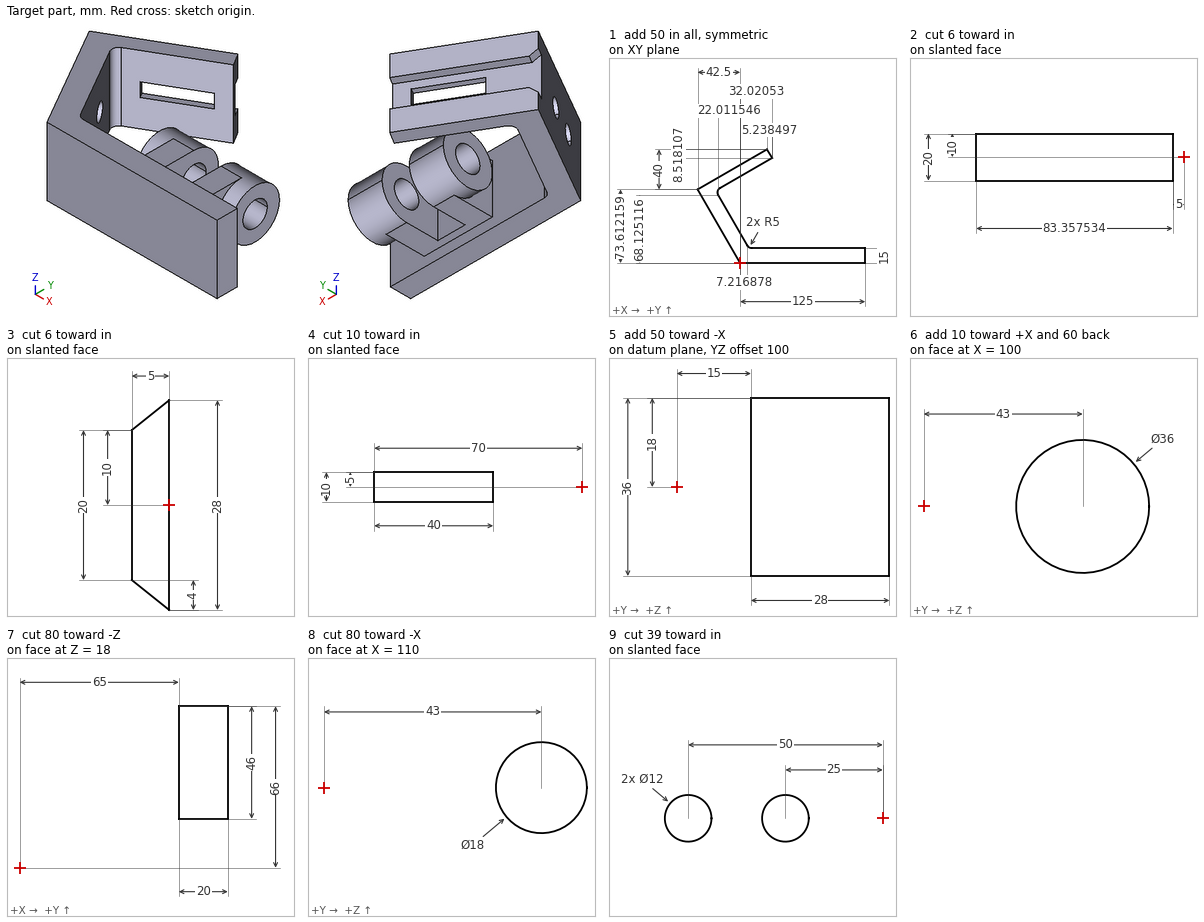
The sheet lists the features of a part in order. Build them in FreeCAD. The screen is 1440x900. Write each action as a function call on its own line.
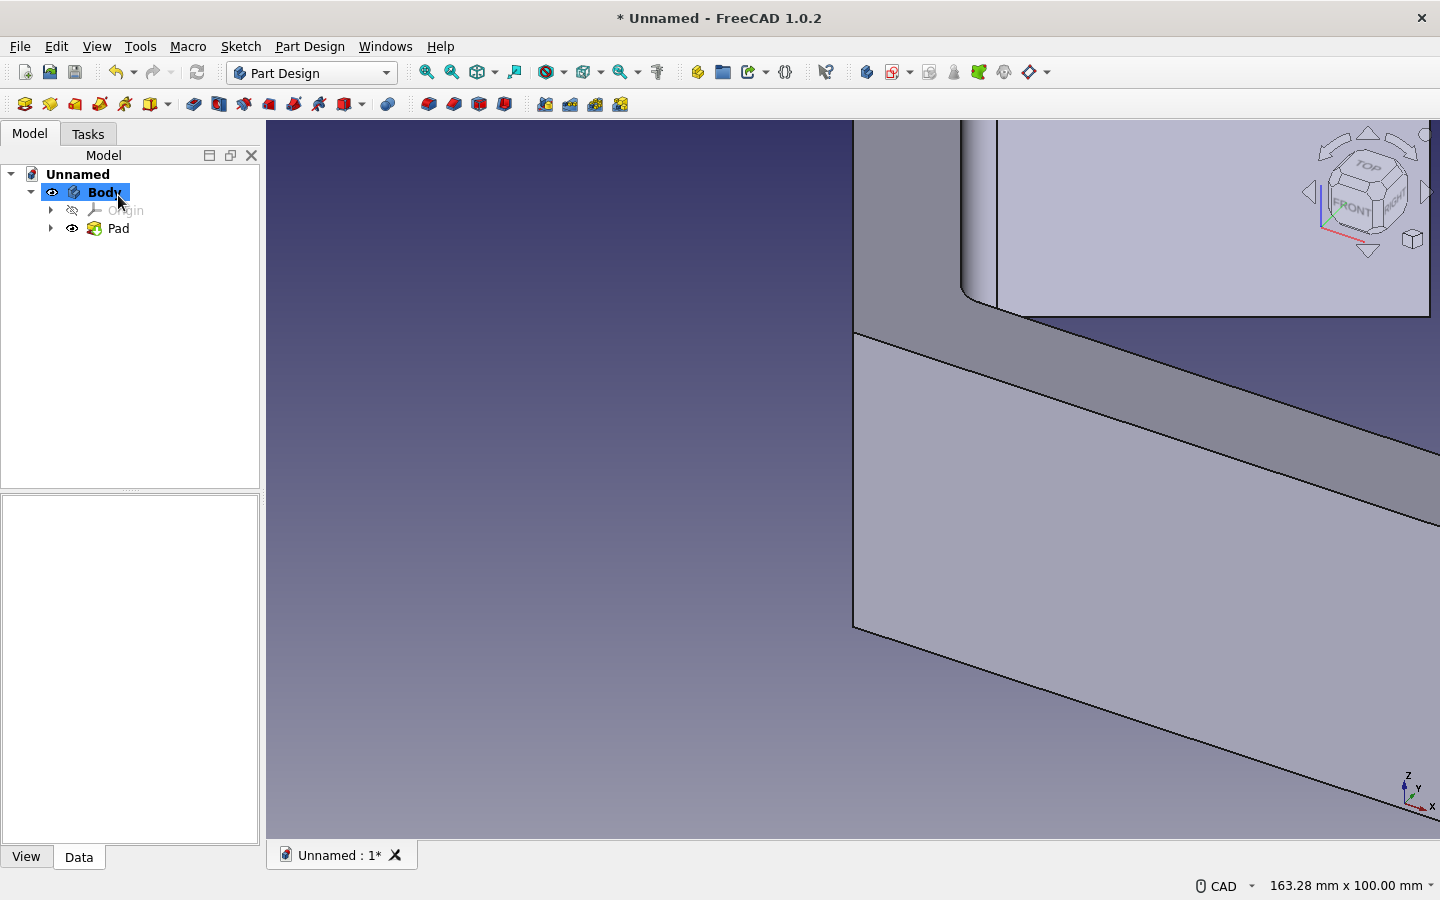
key(v)
key(f)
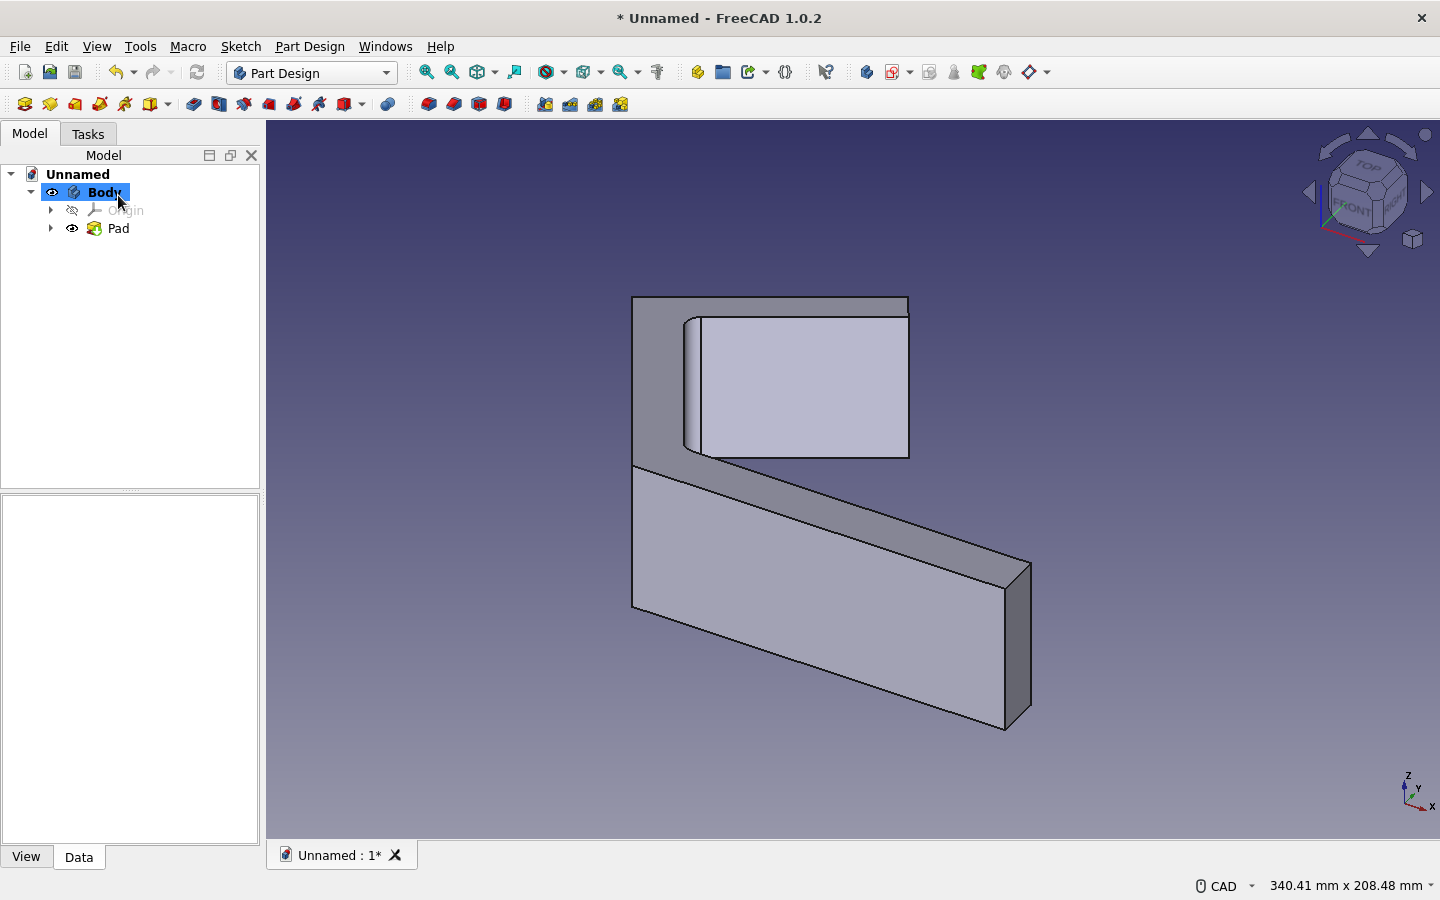
key(4)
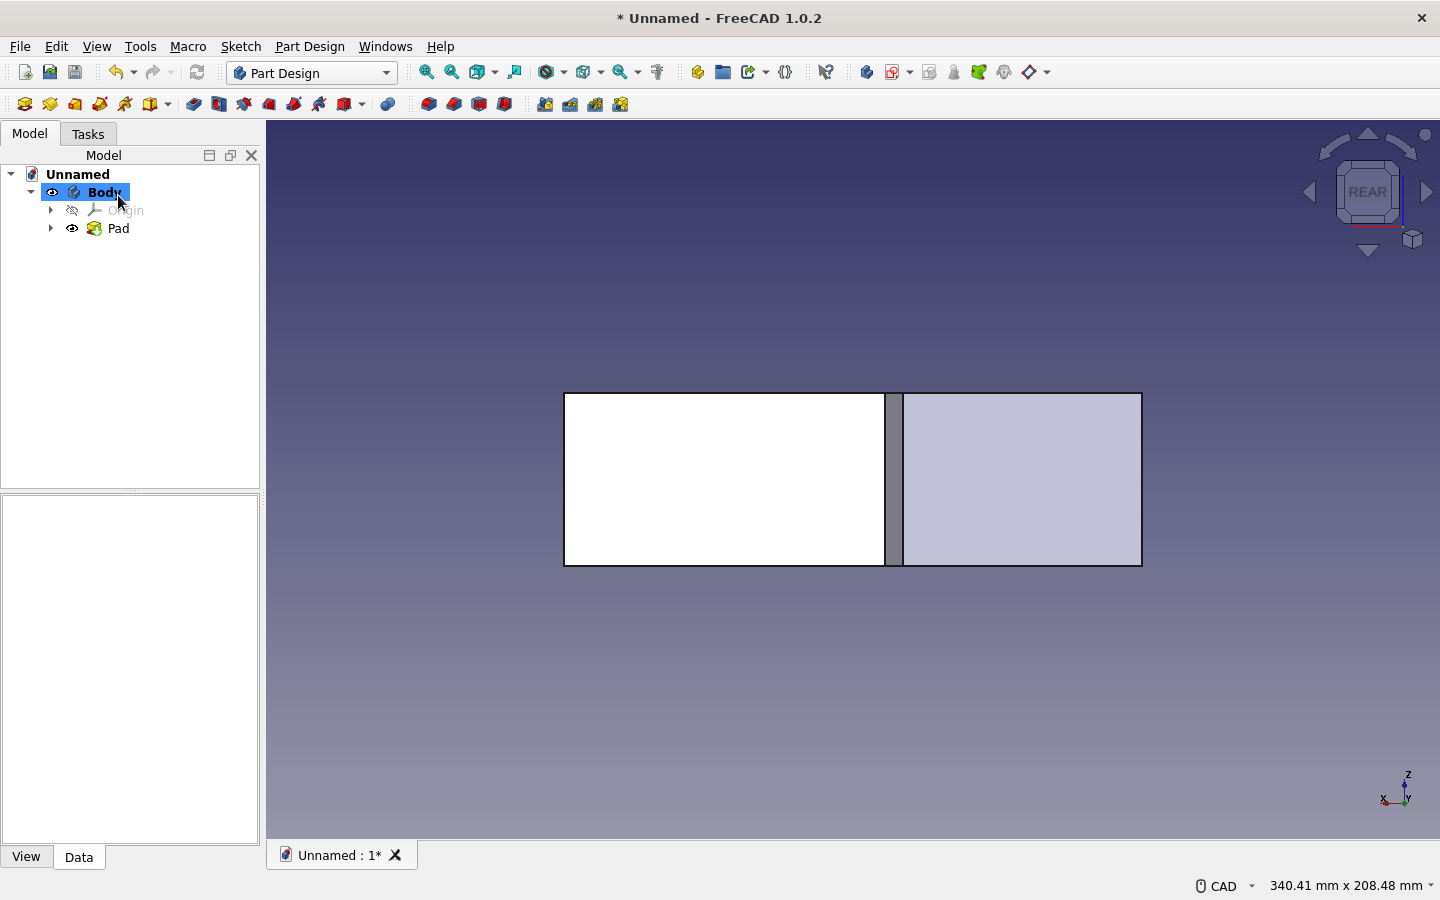
click(988, 478)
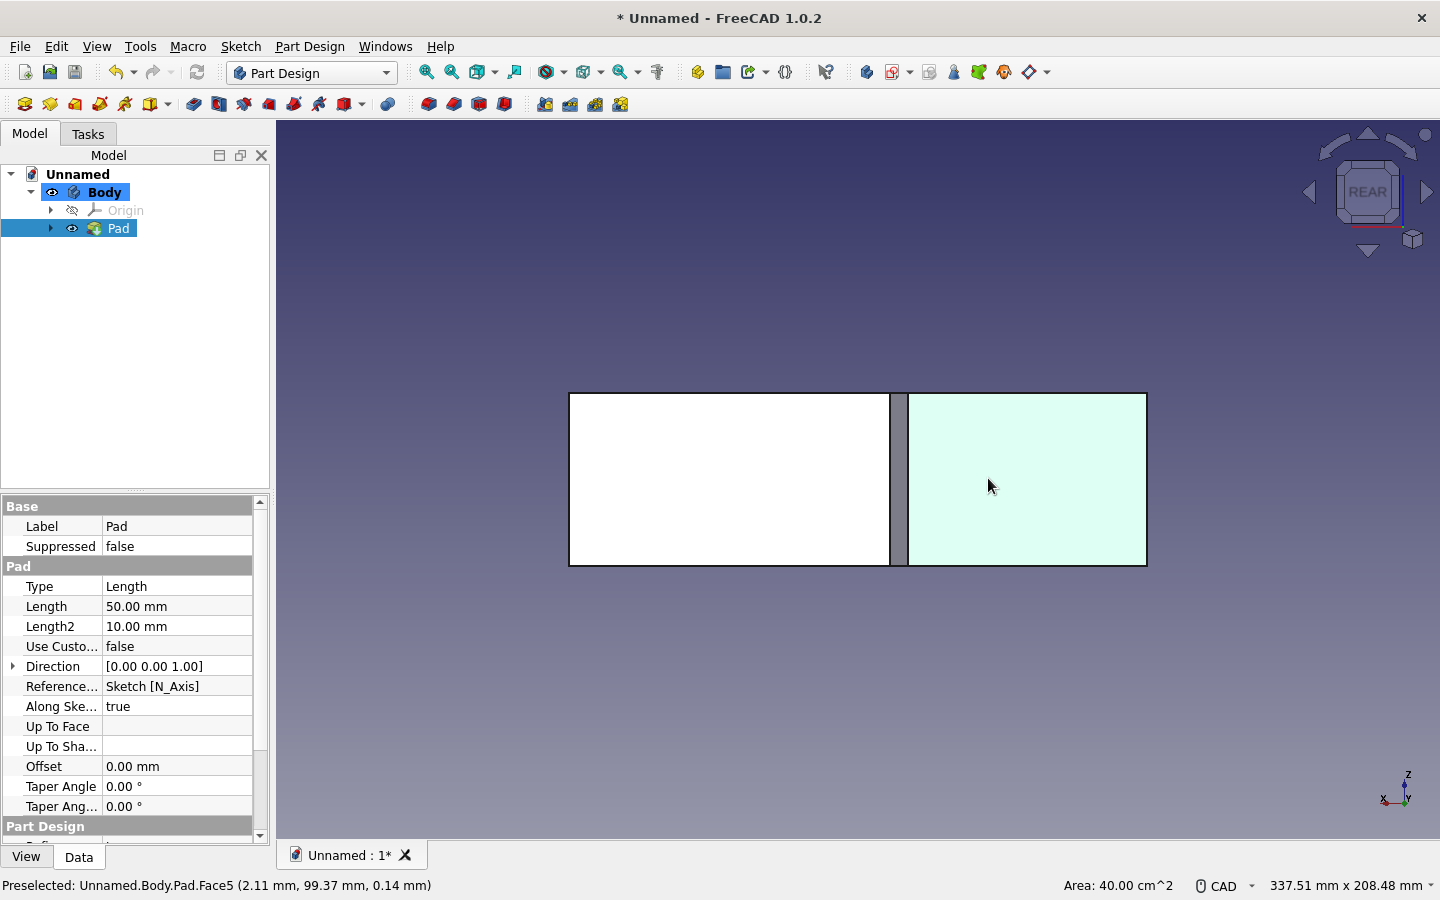
click(892, 72)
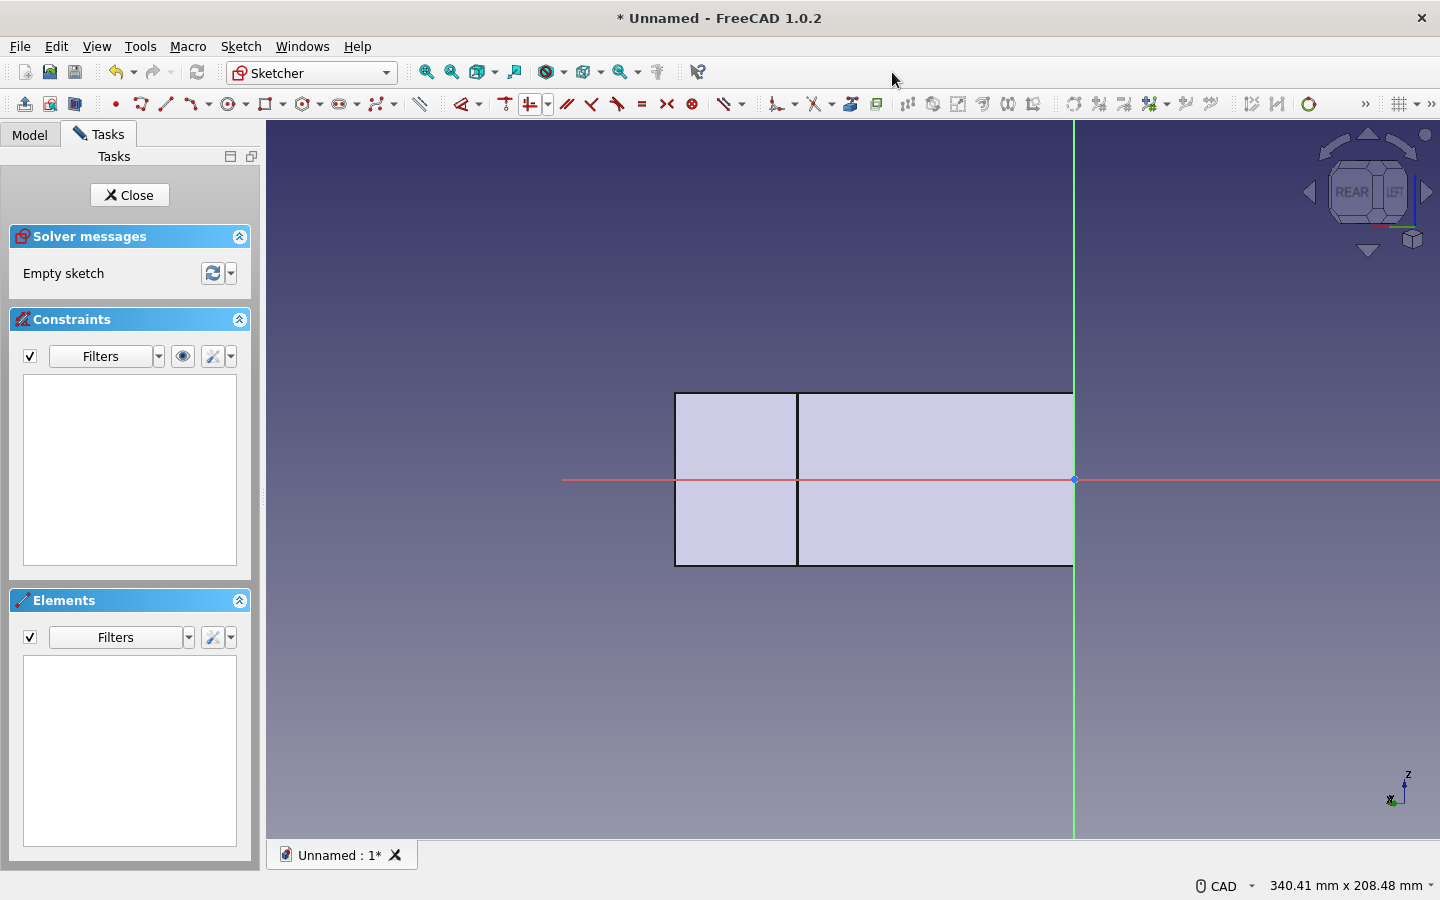
key(q)
key(s)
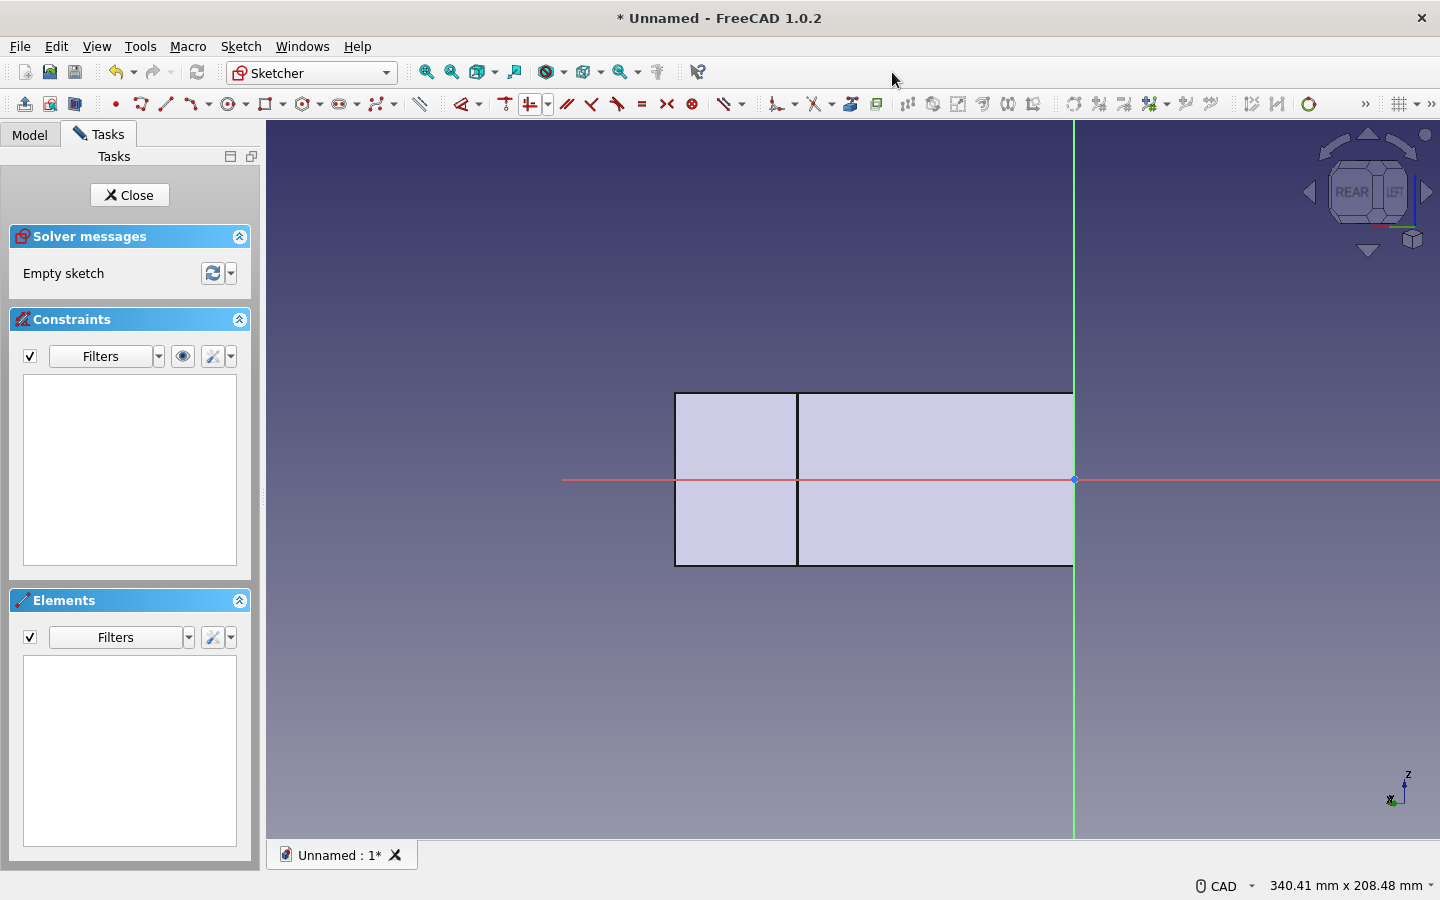
scroll(1034, 479, up, 4)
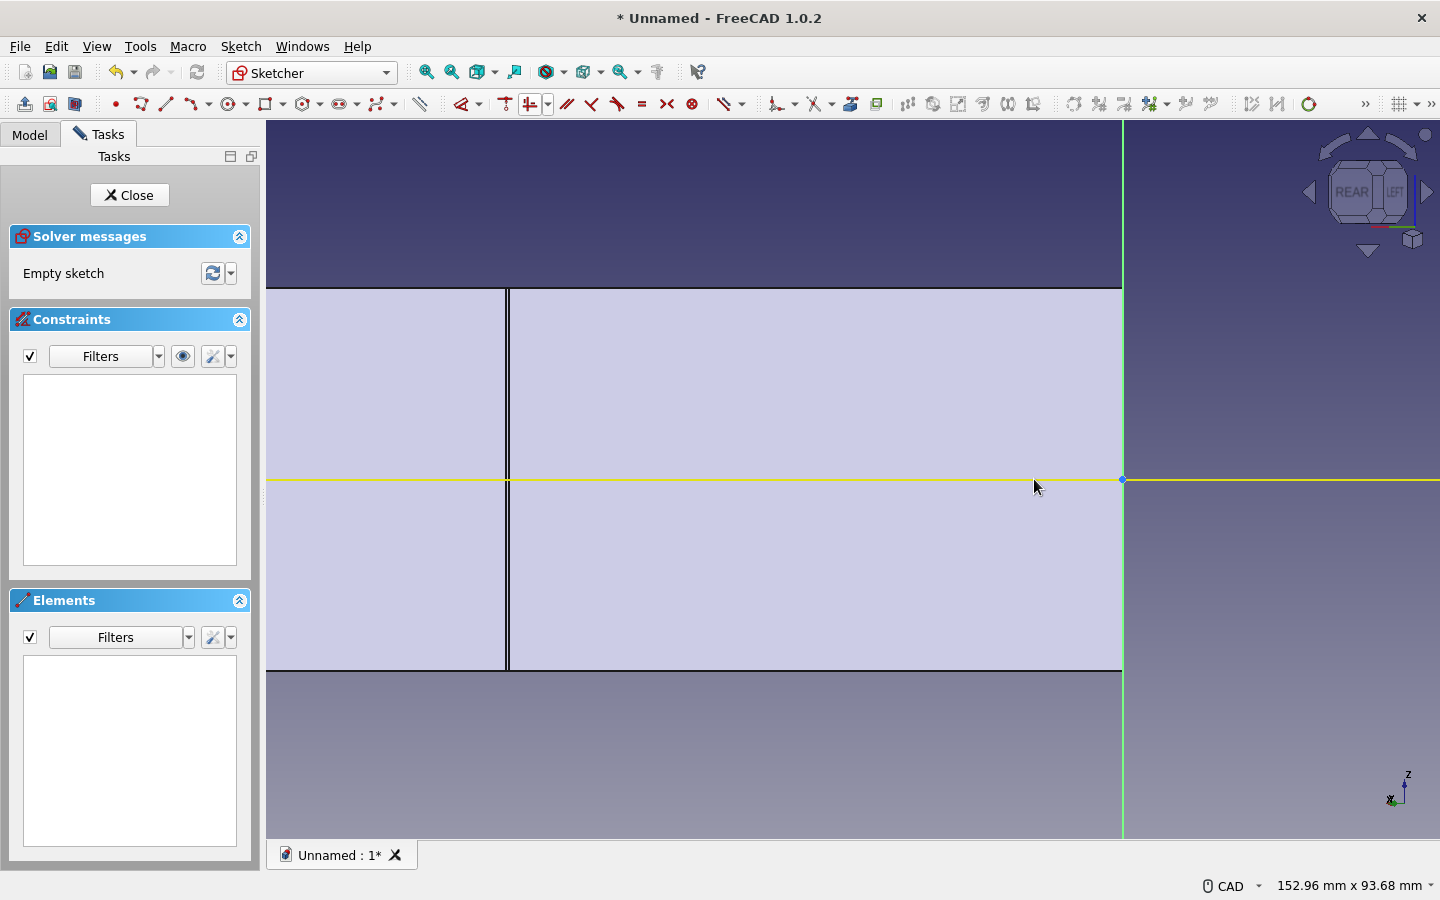
click(264, 104)